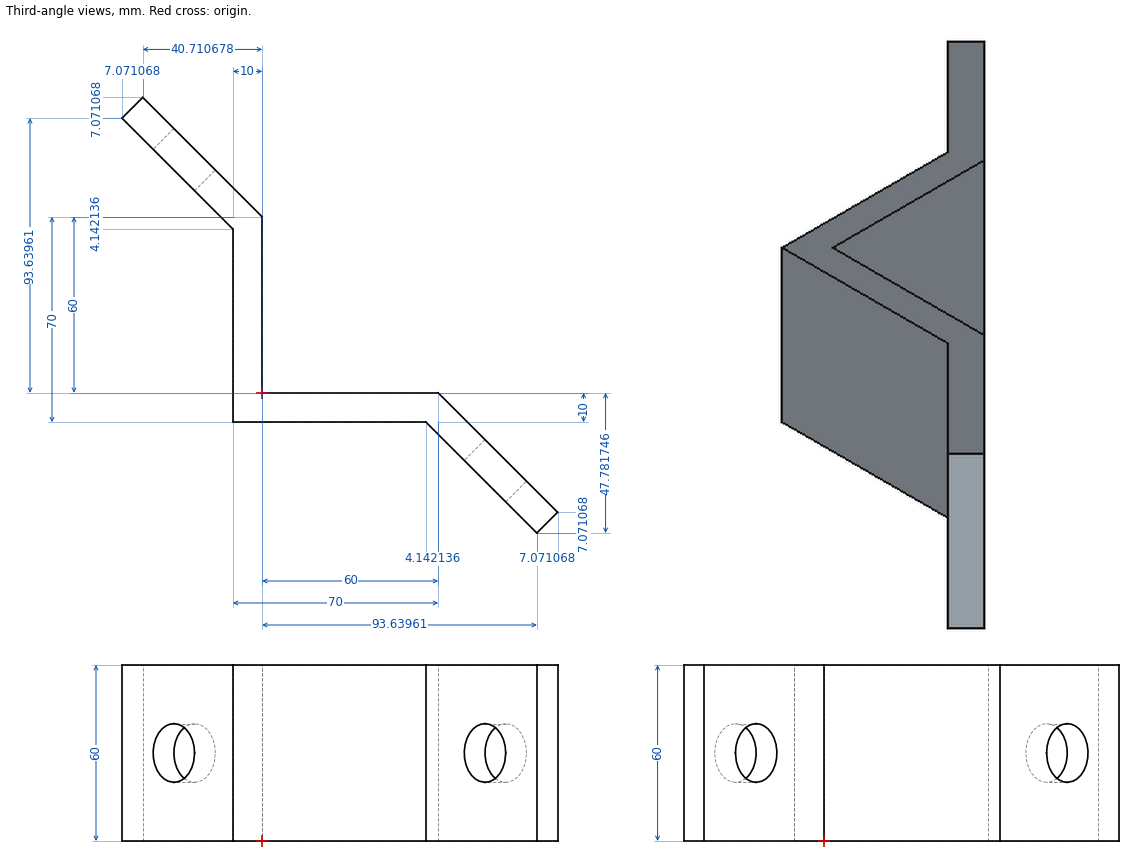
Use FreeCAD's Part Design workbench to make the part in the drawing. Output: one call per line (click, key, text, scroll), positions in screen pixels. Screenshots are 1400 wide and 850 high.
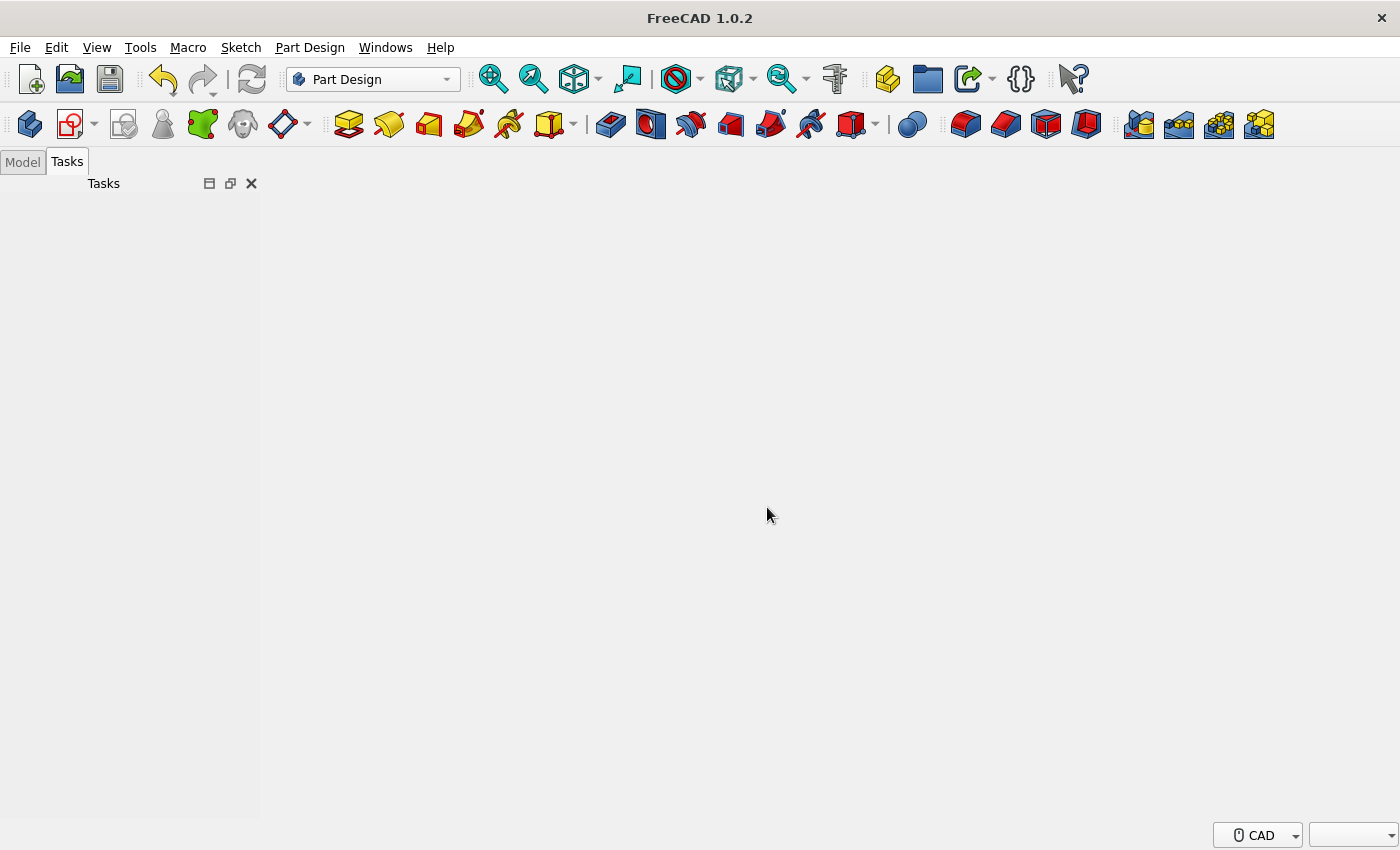
key(ctrl+n)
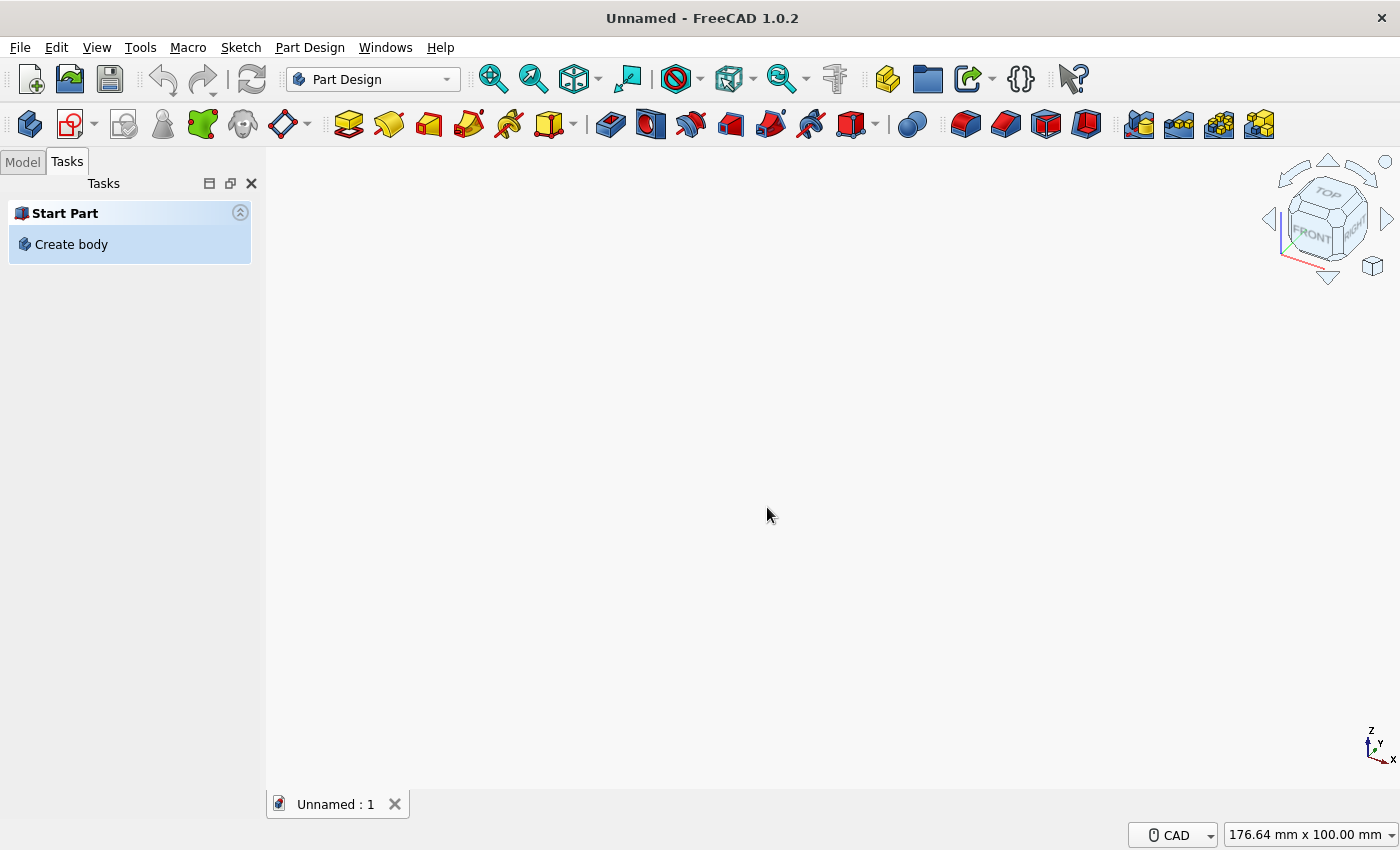
click(70, 124)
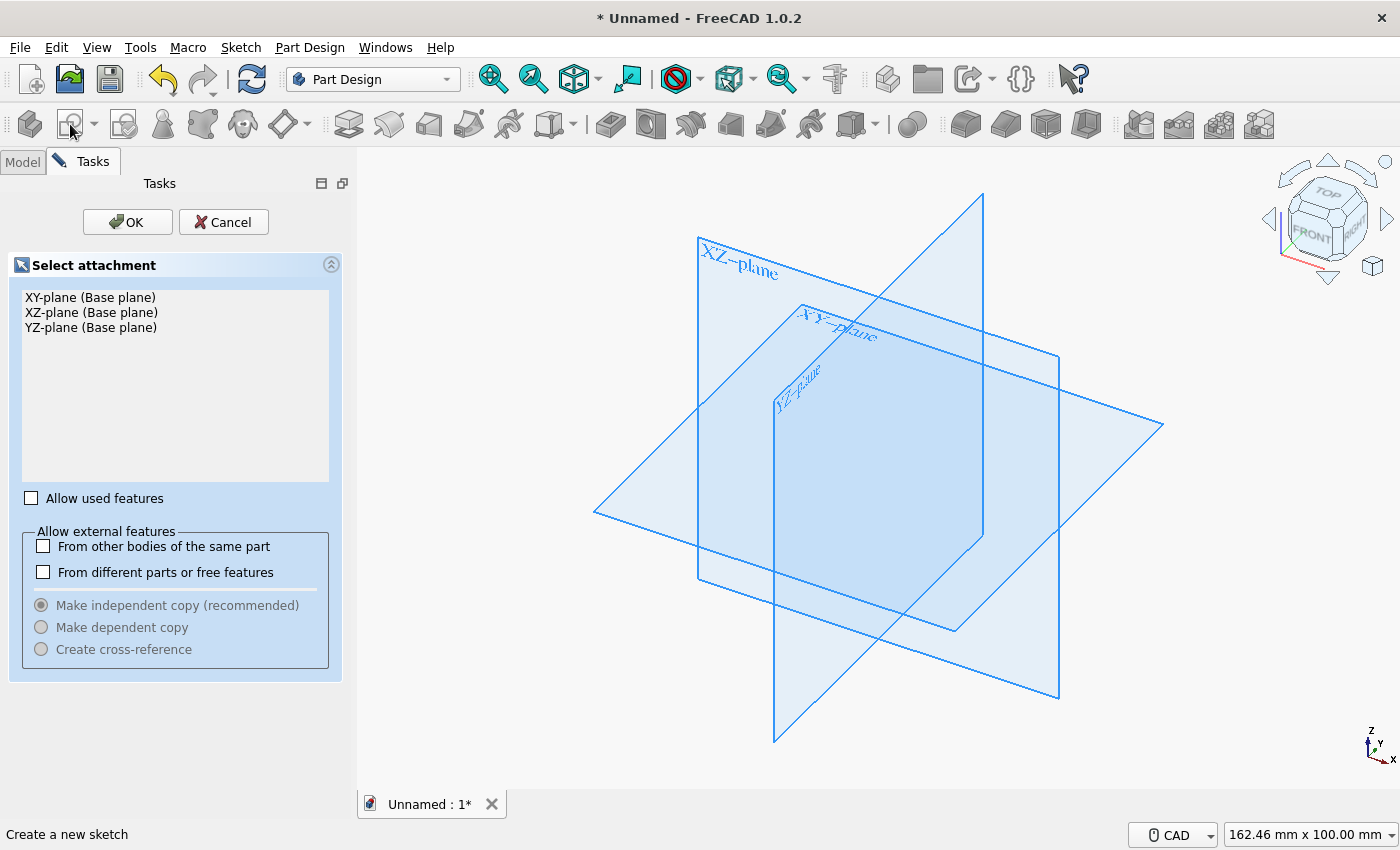
click(82, 298)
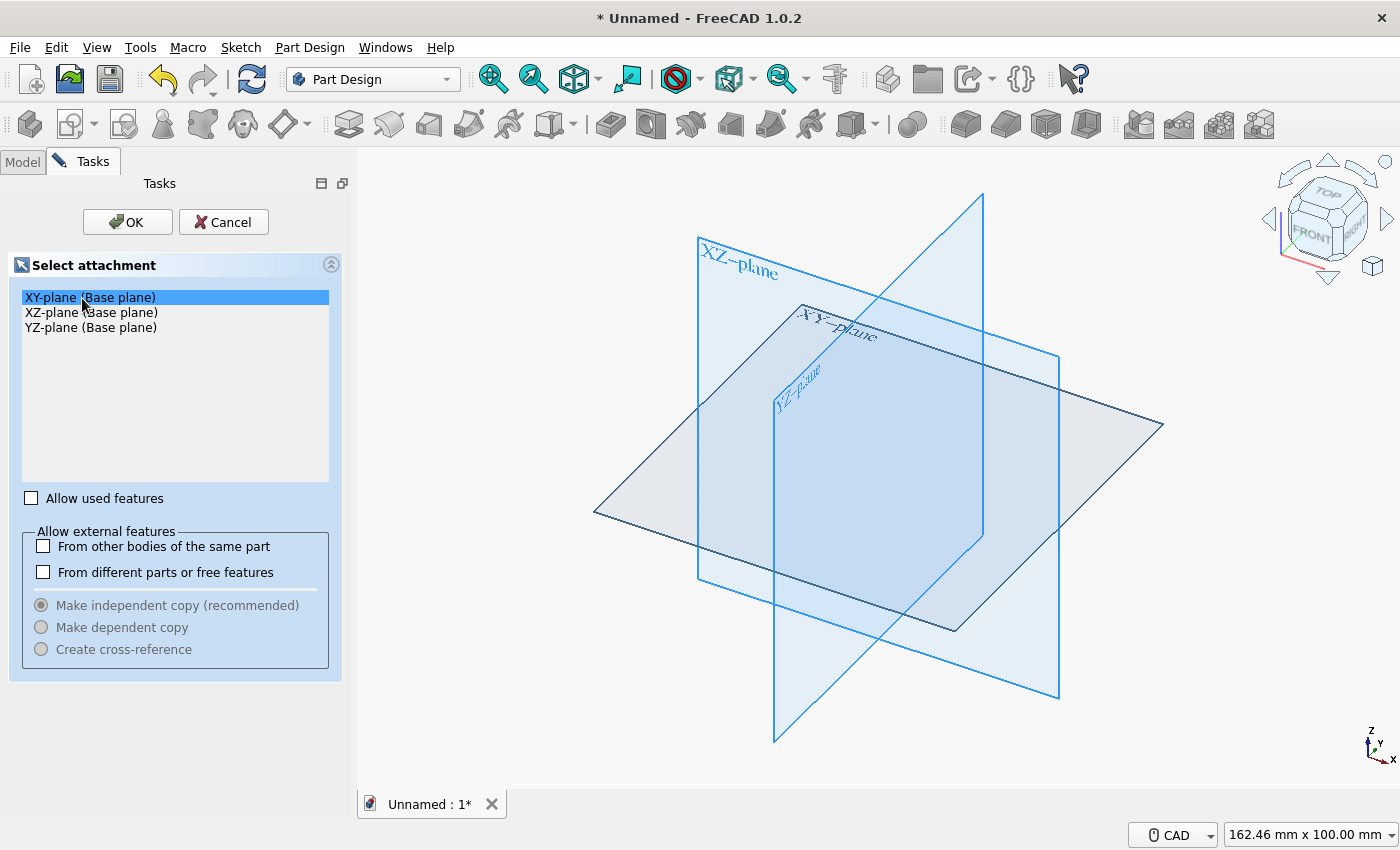
click(128, 222)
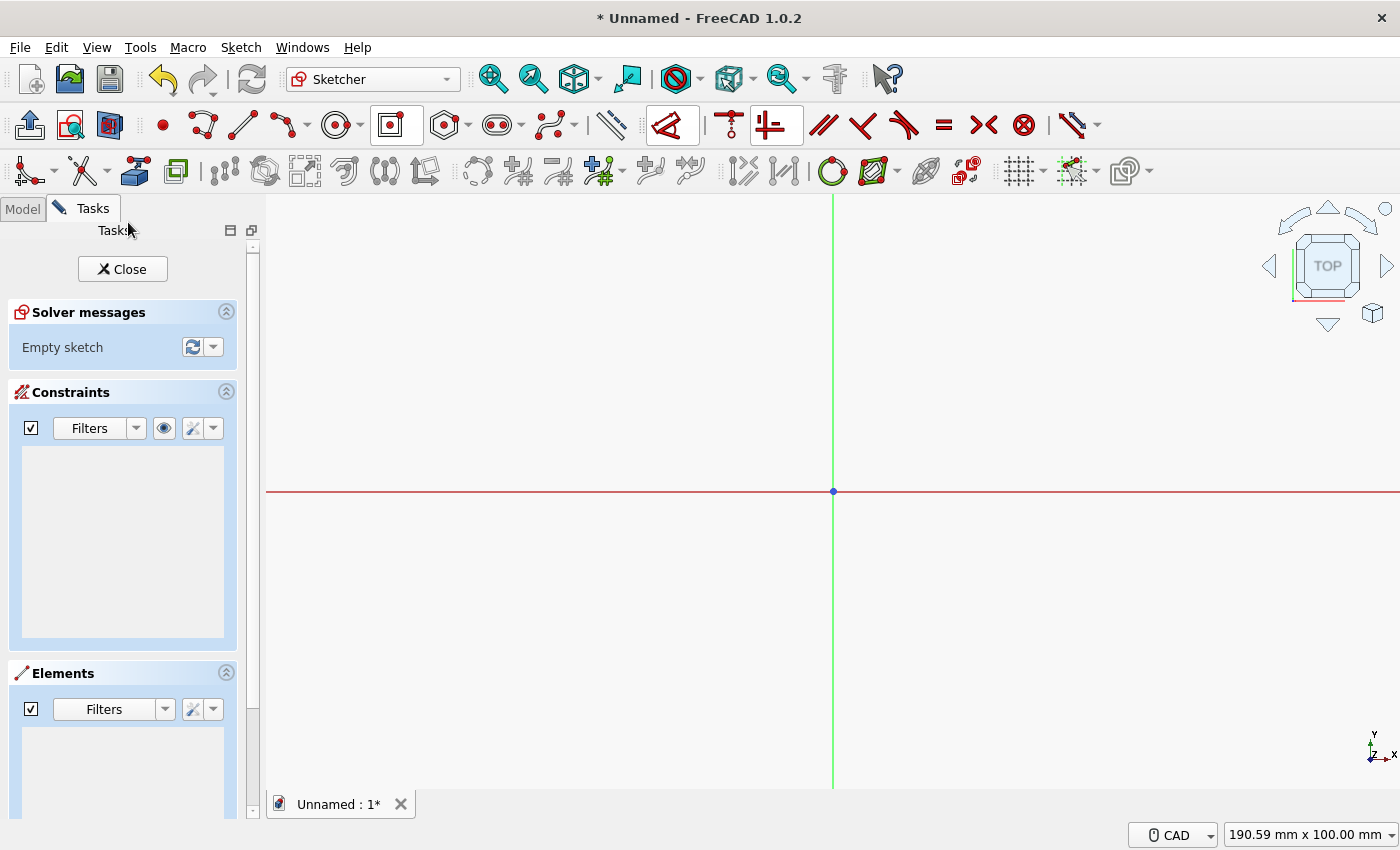
scroll(294, 761, down, 1)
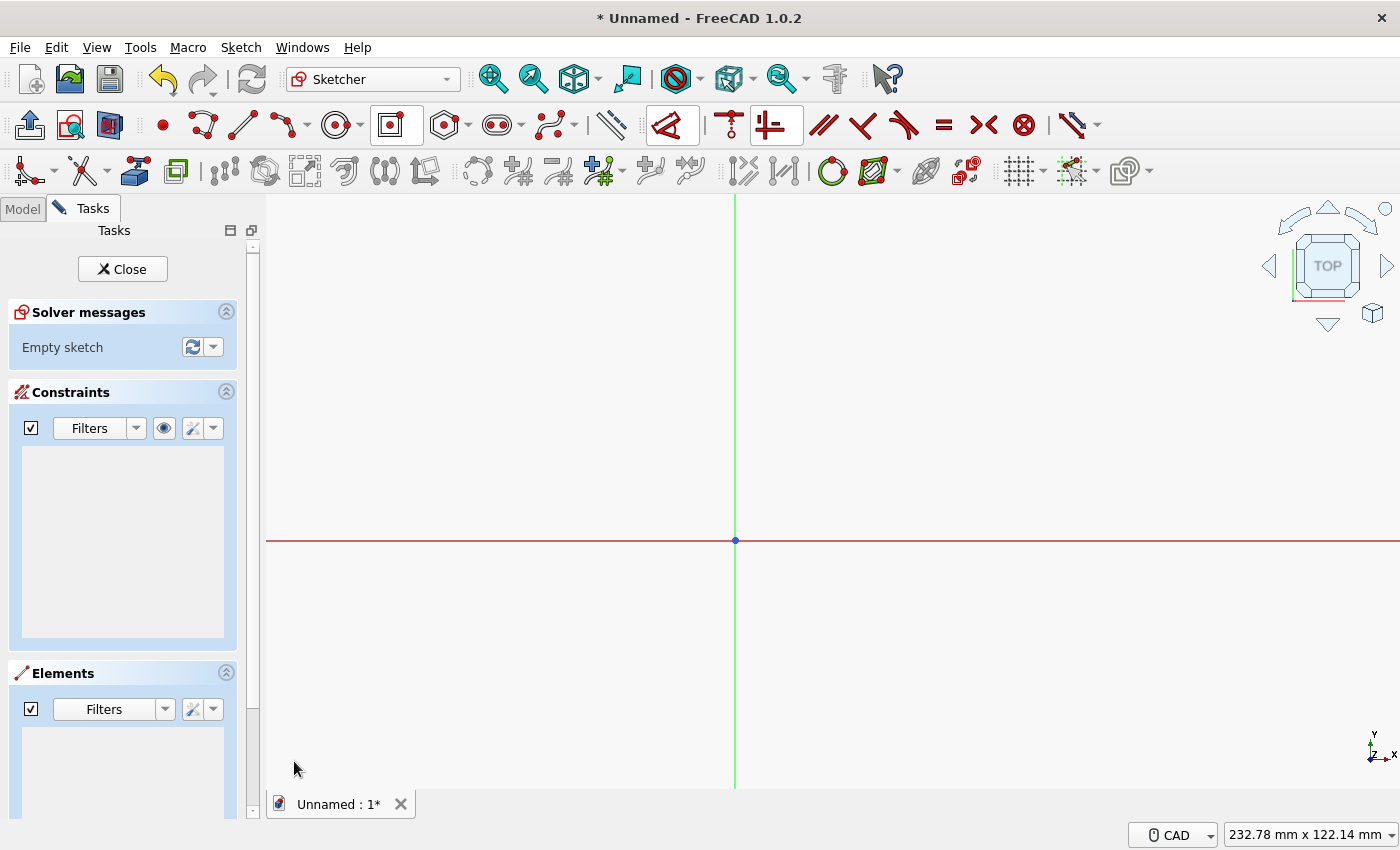
key(g)
key(m)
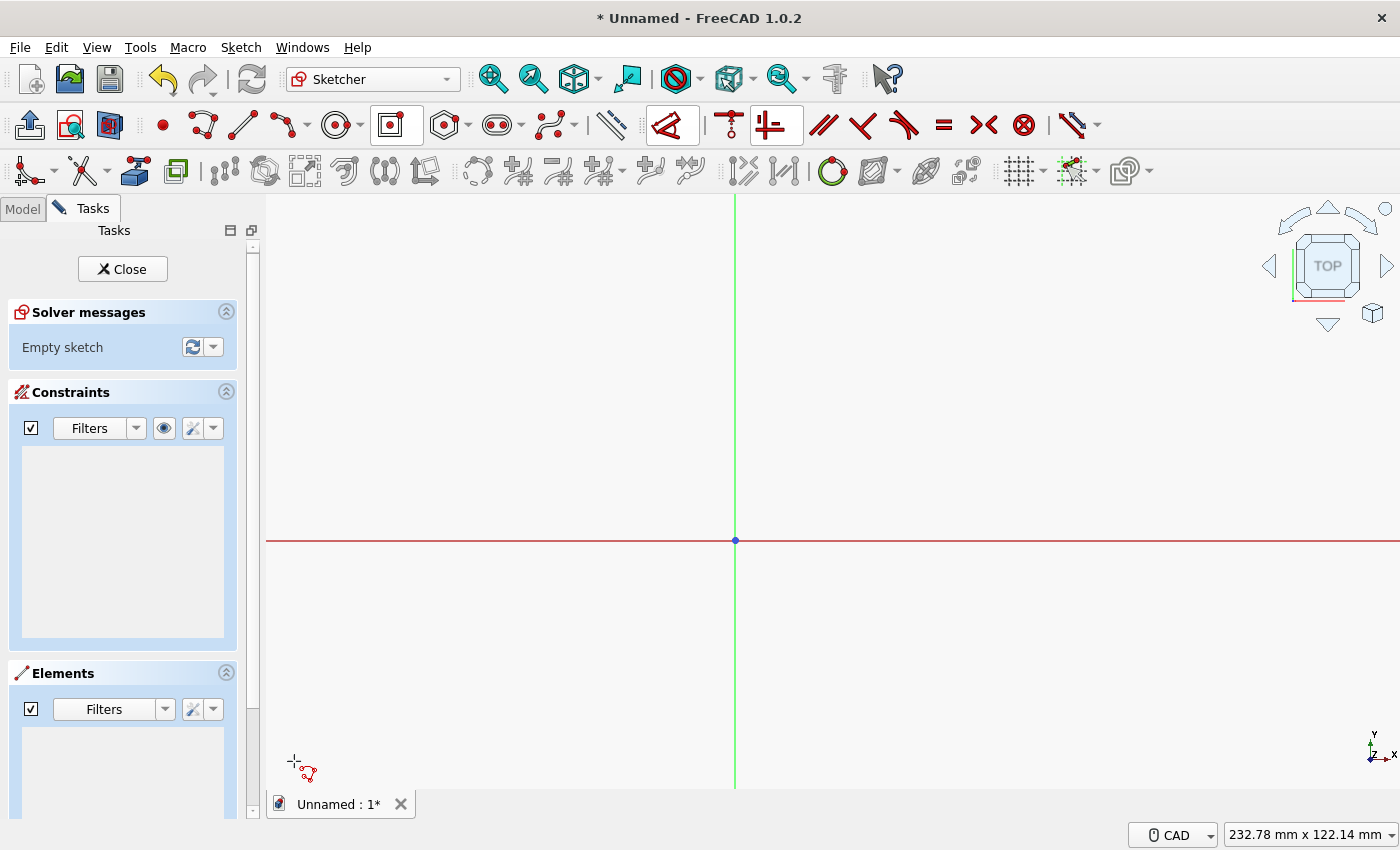
click(735, 541)
click(744, 248)
click(687, 248)
click(687, 589)
click(1028, 589)
click(1028, 532)
click(735, 541)
key(Escape)
key(Escape)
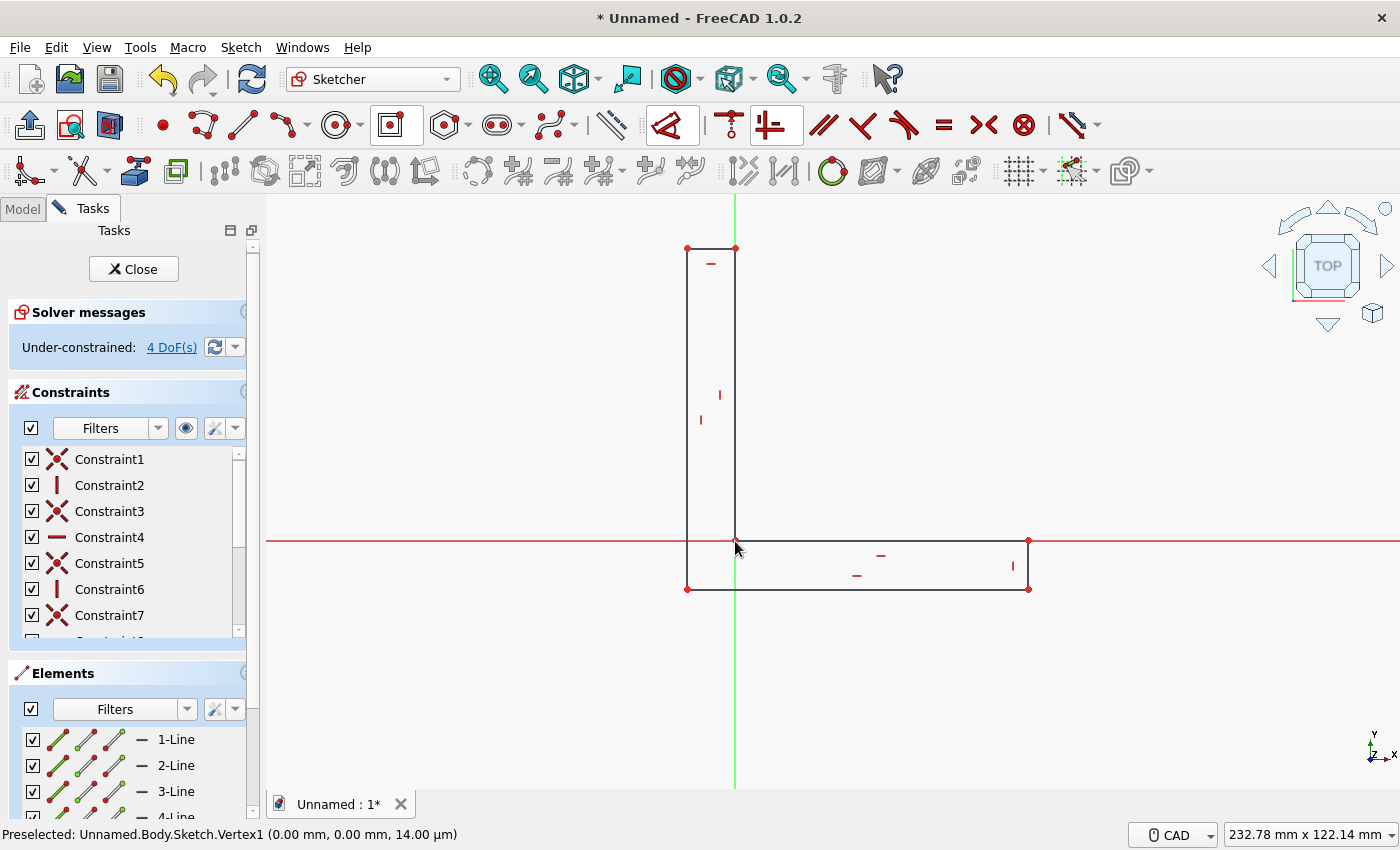
click(666, 126)